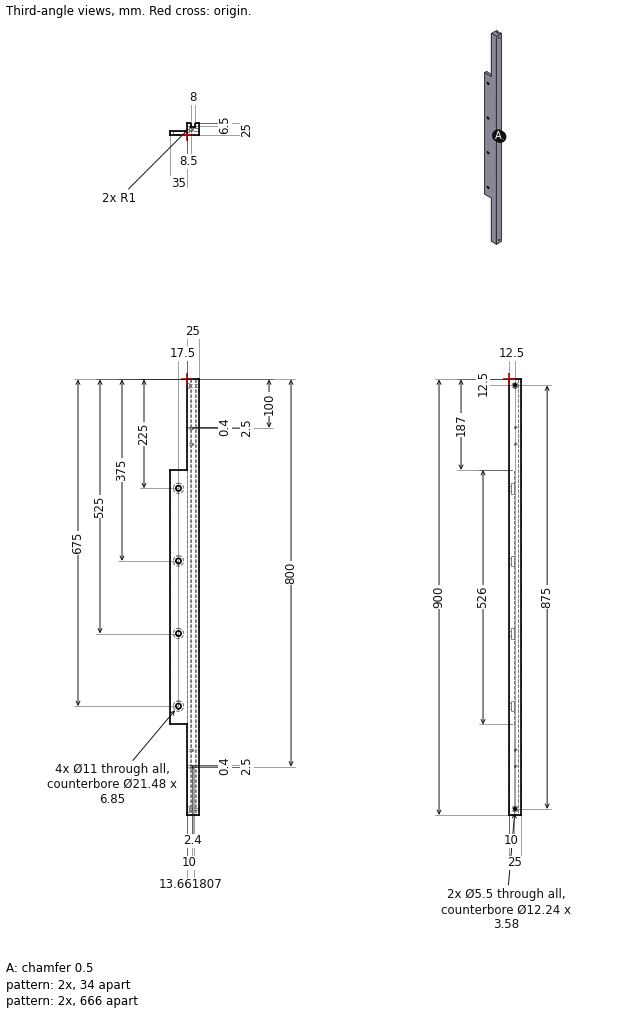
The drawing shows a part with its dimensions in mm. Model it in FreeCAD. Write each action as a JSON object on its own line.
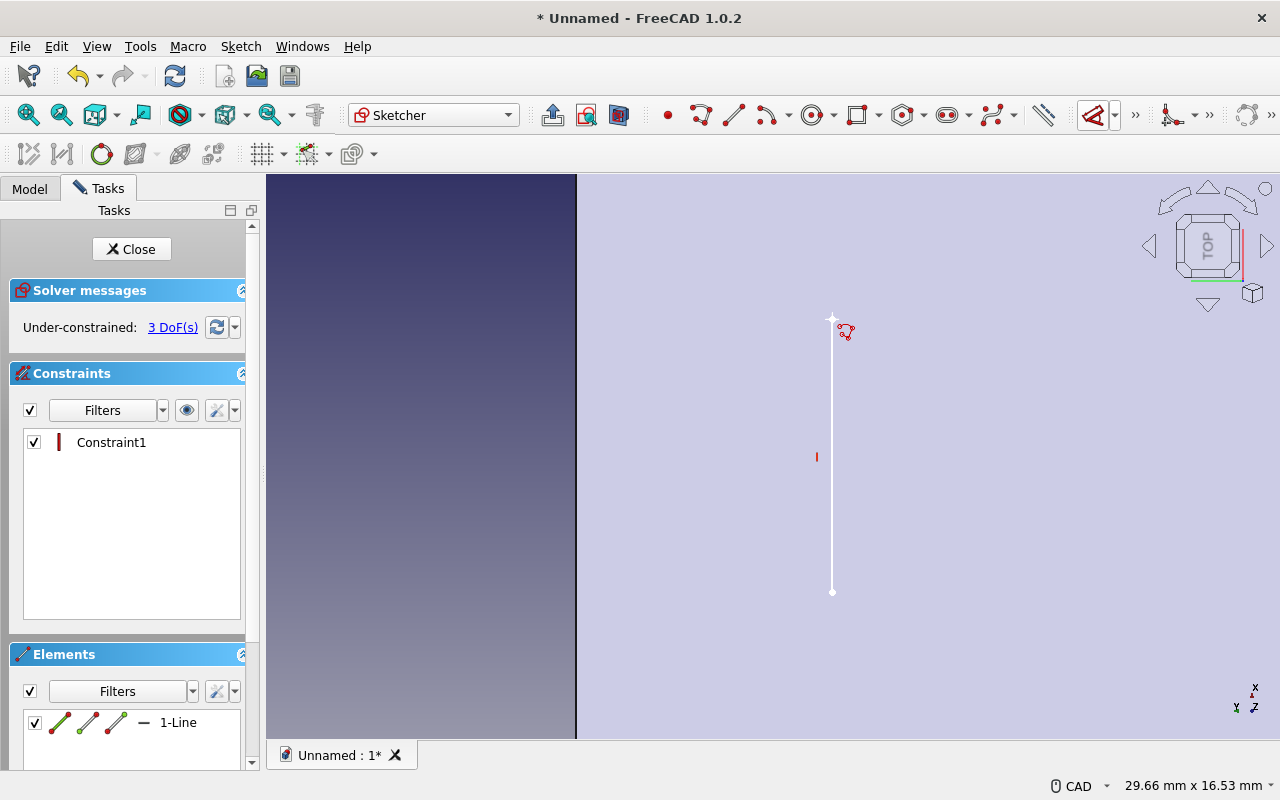
{"action": "left_click", "coordinate": [798, 285]}
{"action": "left_click", "coordinate": [576, 285]}
{"action": "left_click", "coordinate": [576, 627]}
{"action": "left_click", "coordinate": [798, 627]}
{"action": "right_click", "coordinate": [798, 627]}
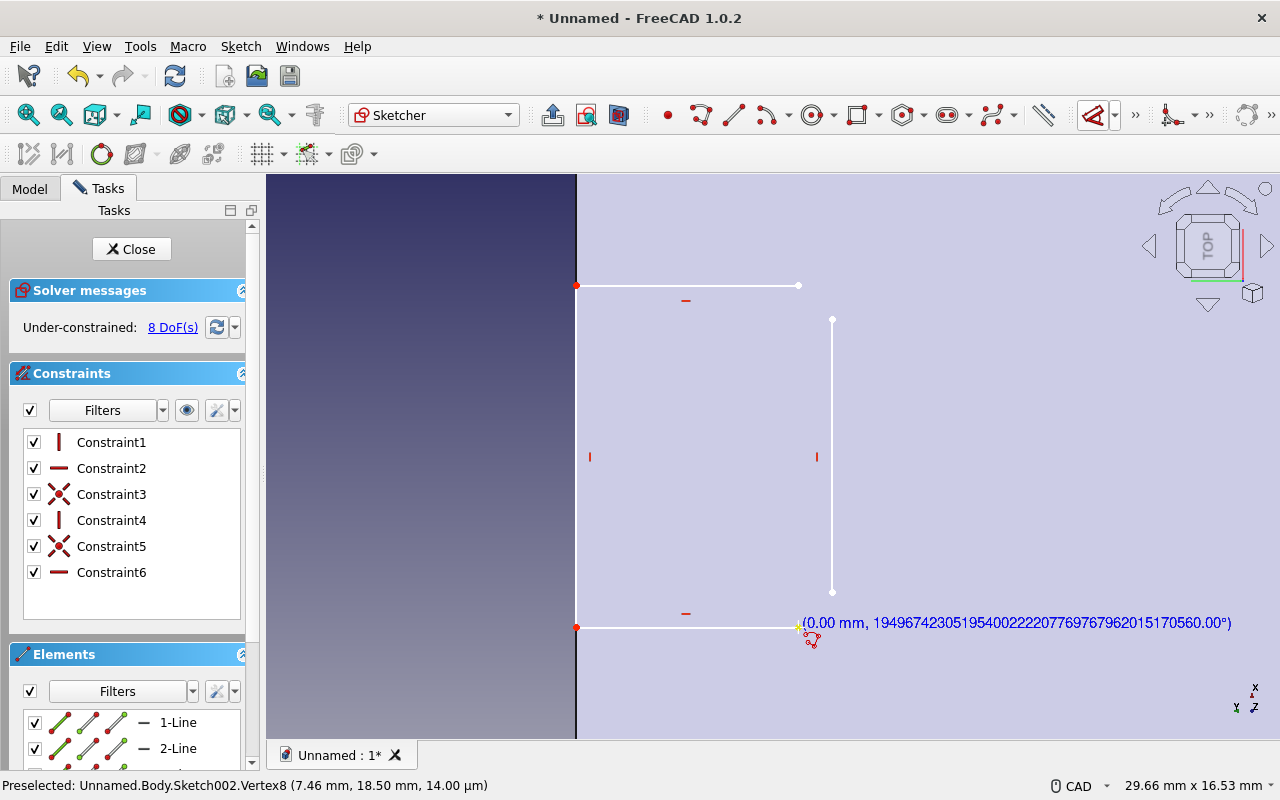
{"action": "left_click", "coordinate": [788, 116]}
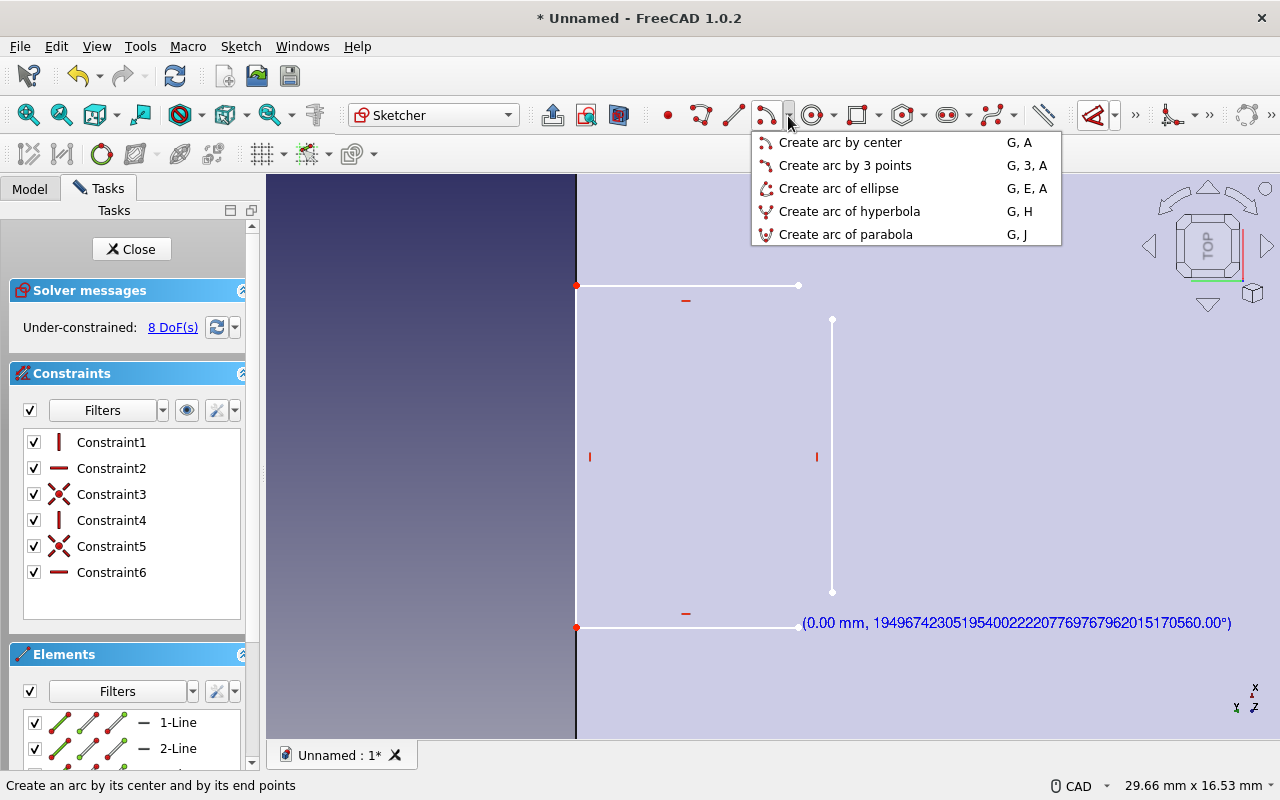
{"action": "left_click", "coordinate": [906, 166]}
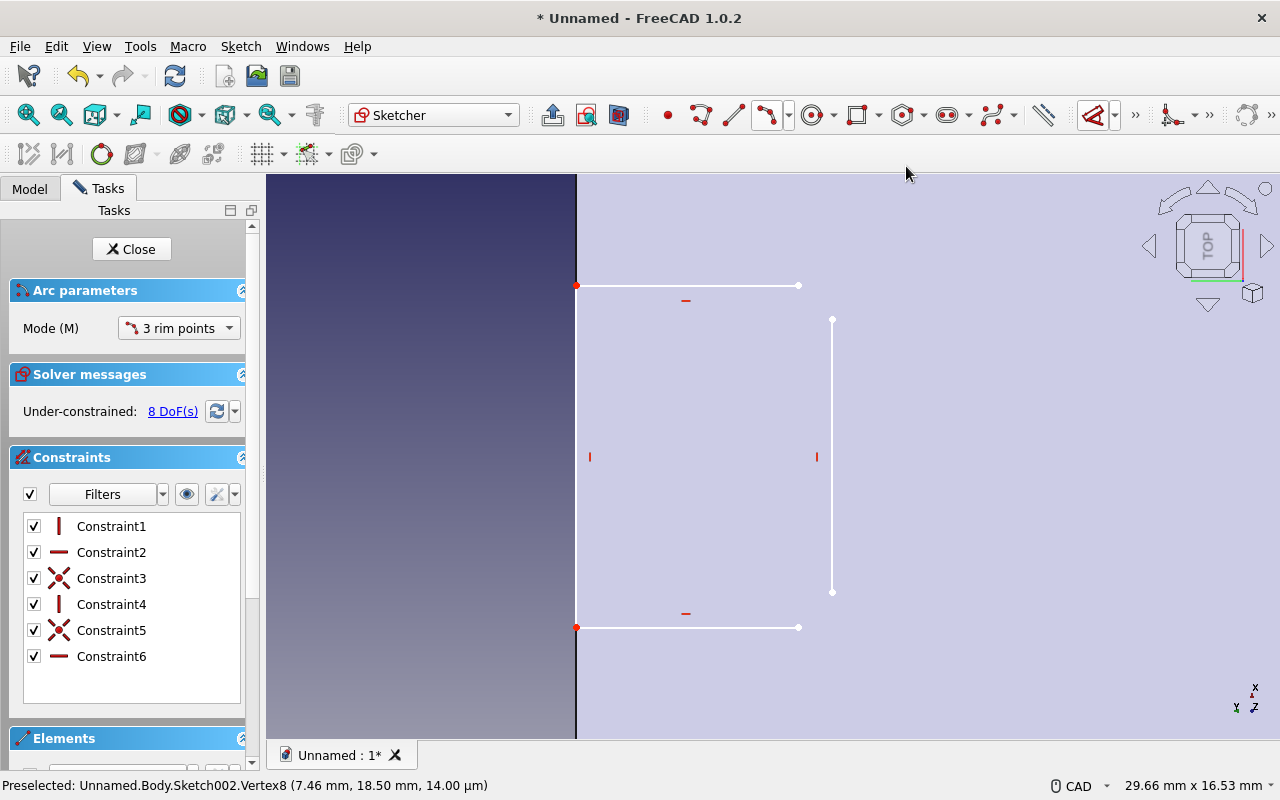
{"action": "left_click", "coordinate": [832, 320]}
{"action": "left_click", "coordinate": [798, 286]}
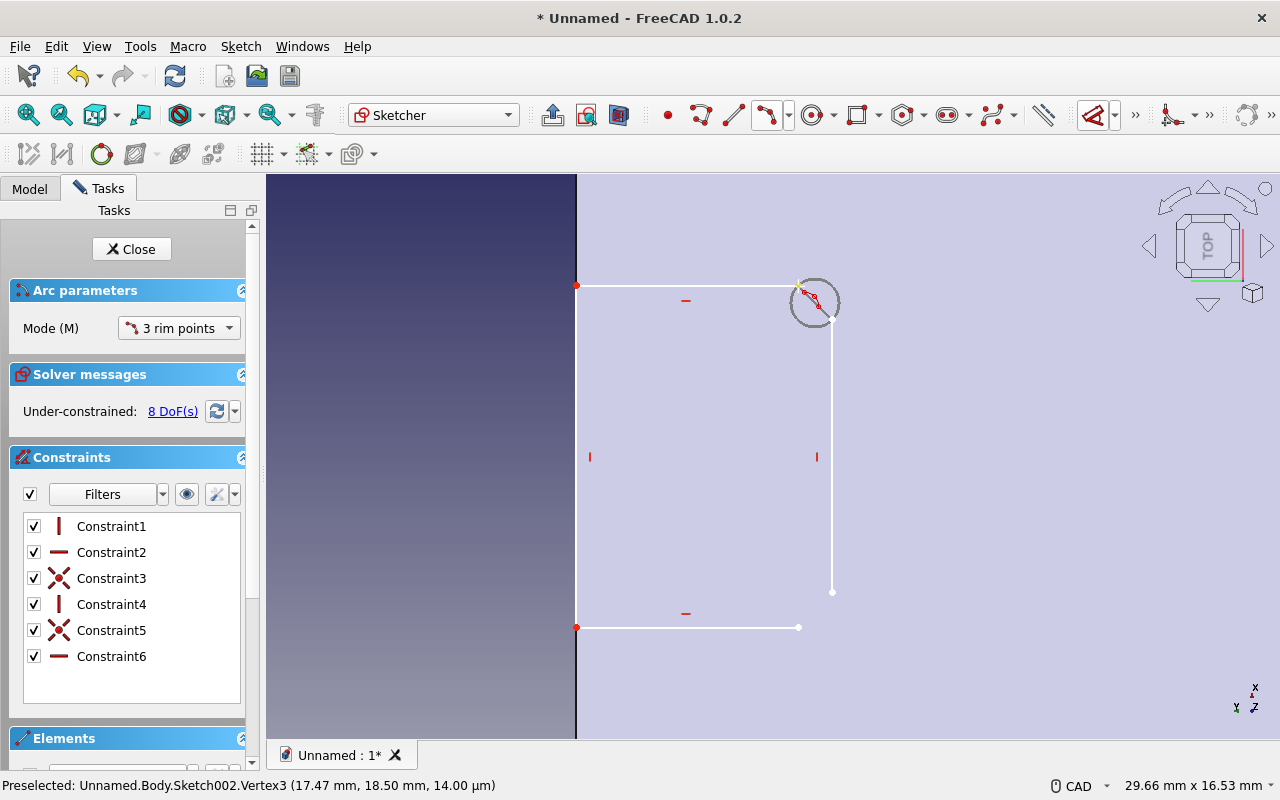
{"action": "scroll", "coordinate": [822, 295], "scroll_direction": "up", "scroll_amount": 3}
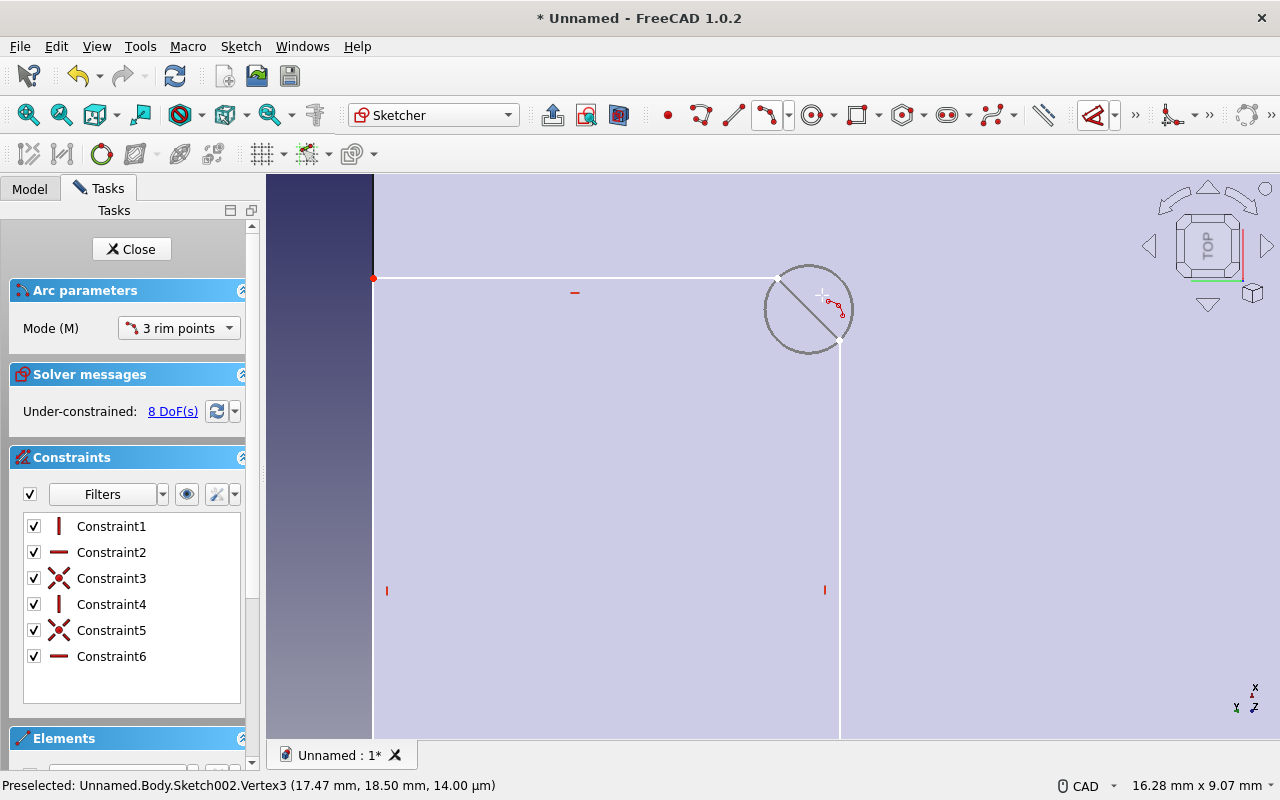
{"action": "left_click", "coordinate": [822, 295]}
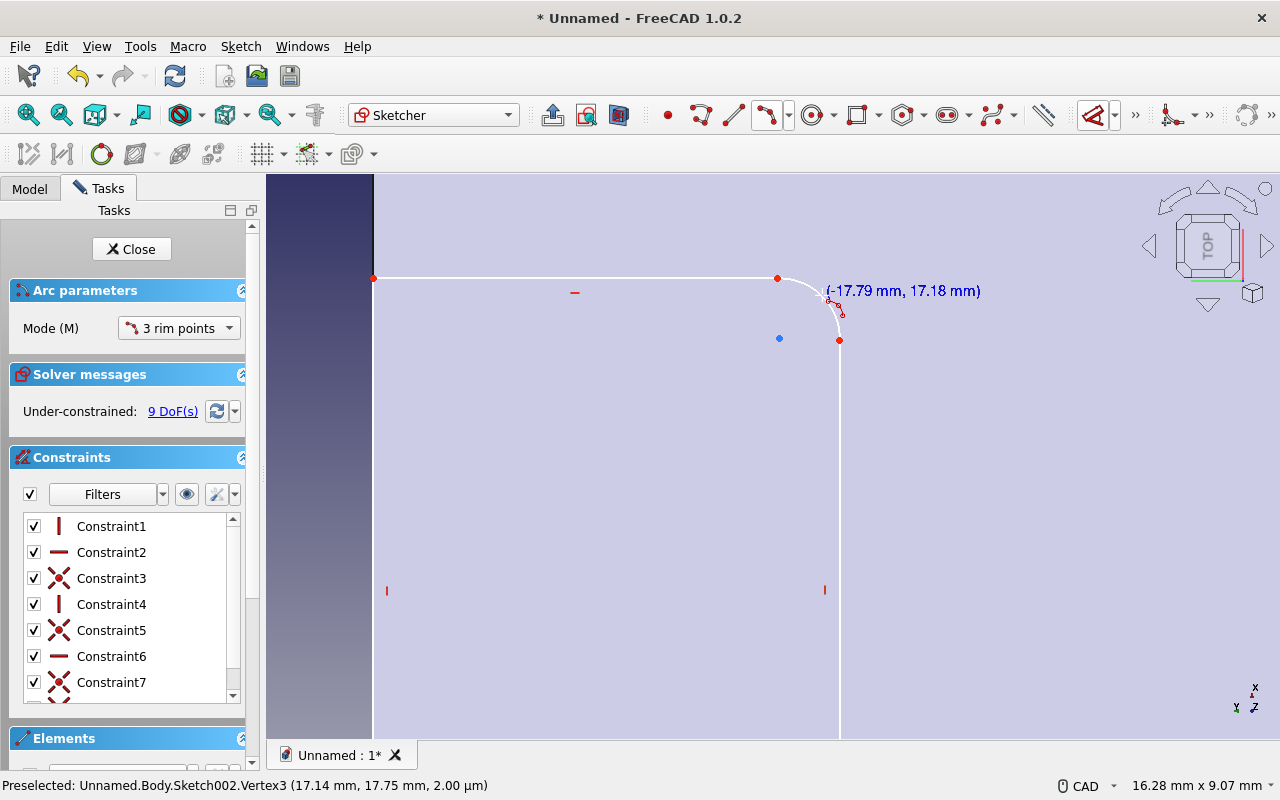
{"action": "scroll", "coordinate": [824, 297], "scroll_direction": "down", "scroll_amount": 3}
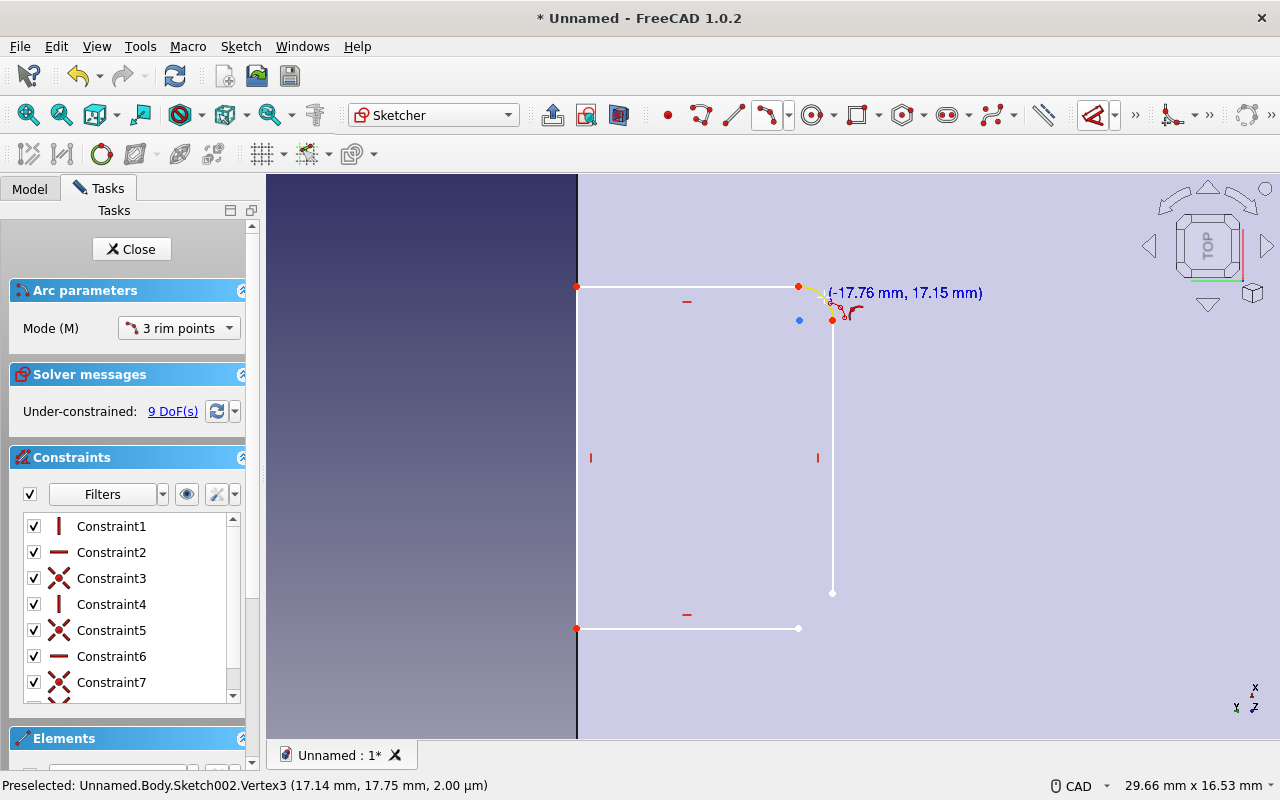
{"action": "left_click", "coordinate": [799, 629]}
{"action": "left_click", "coordinate": [833, 594]}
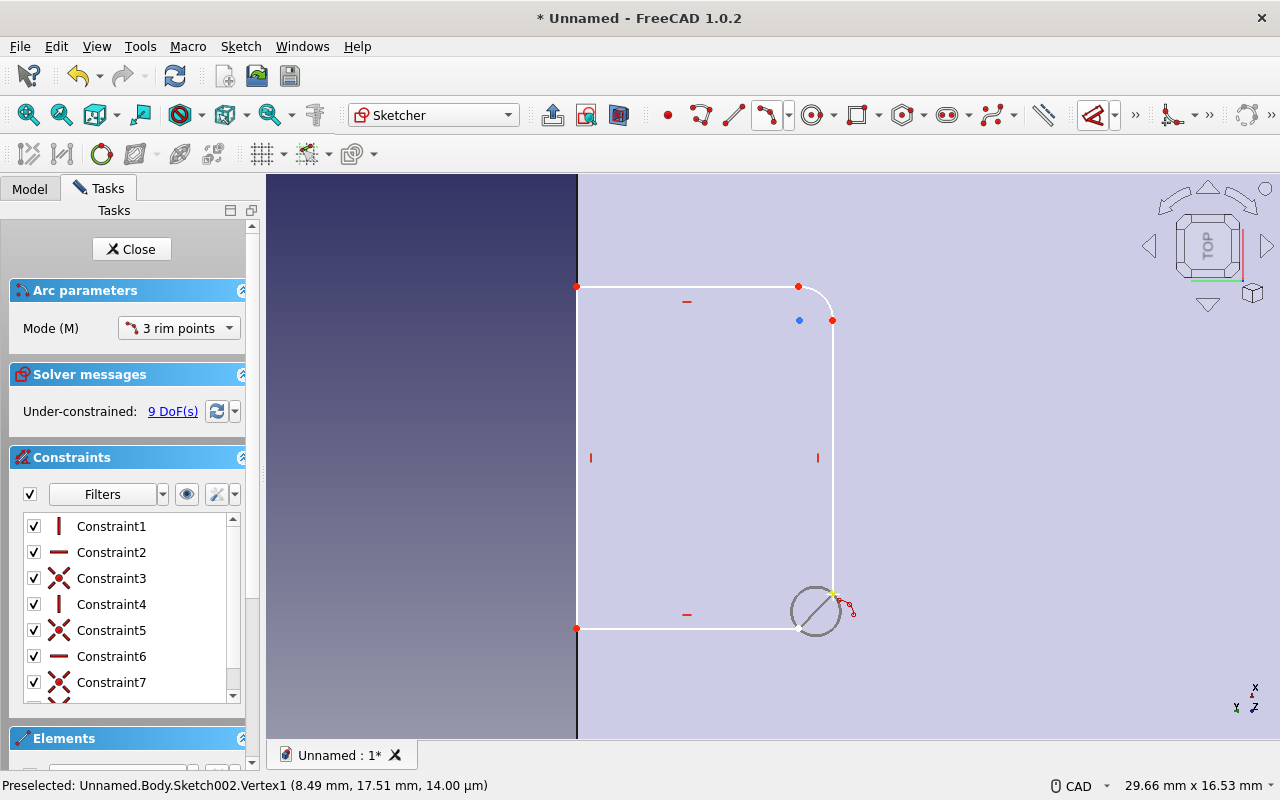
{"action": "scroll", "coordinate": [823, 618], "scroll_direction": "up", "scroll_amount": 3}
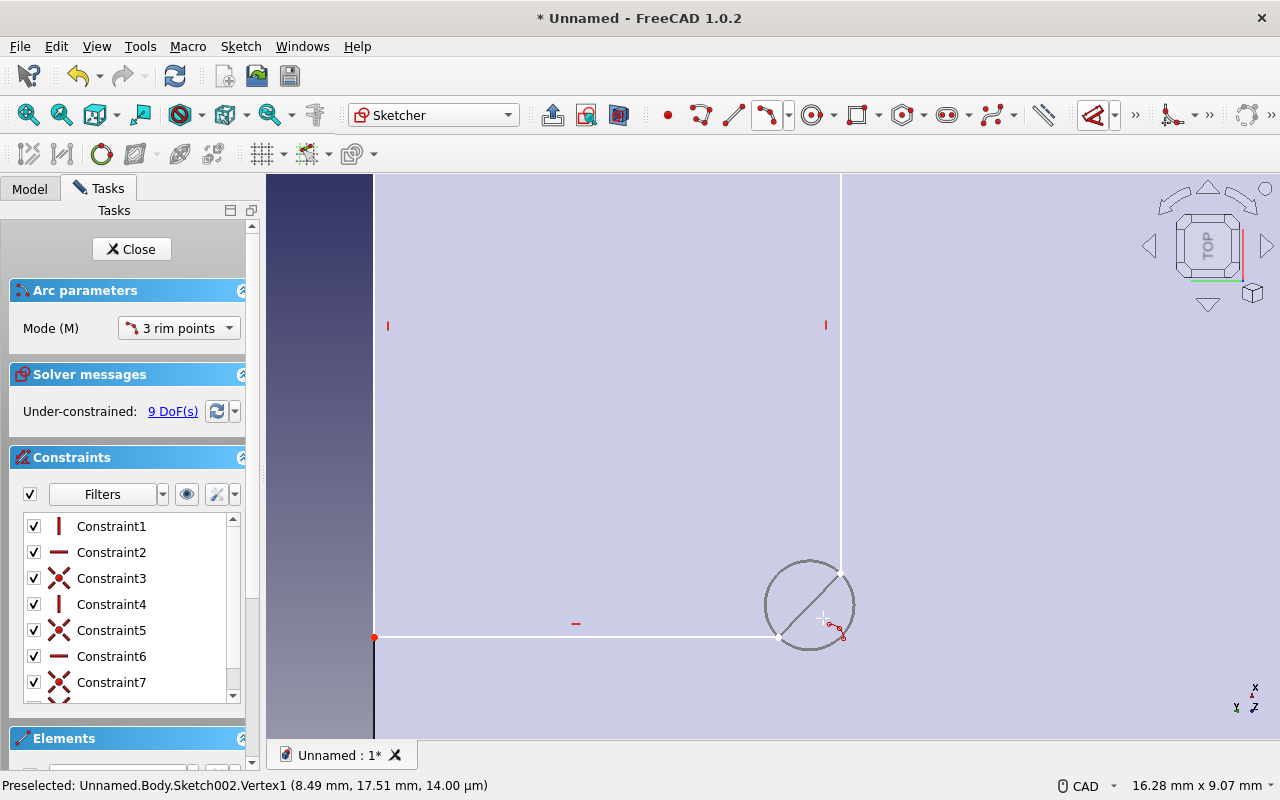
{"action": "left_click", "coordinate": [823, 617]}
{"action": "key", "text": "Escape"}